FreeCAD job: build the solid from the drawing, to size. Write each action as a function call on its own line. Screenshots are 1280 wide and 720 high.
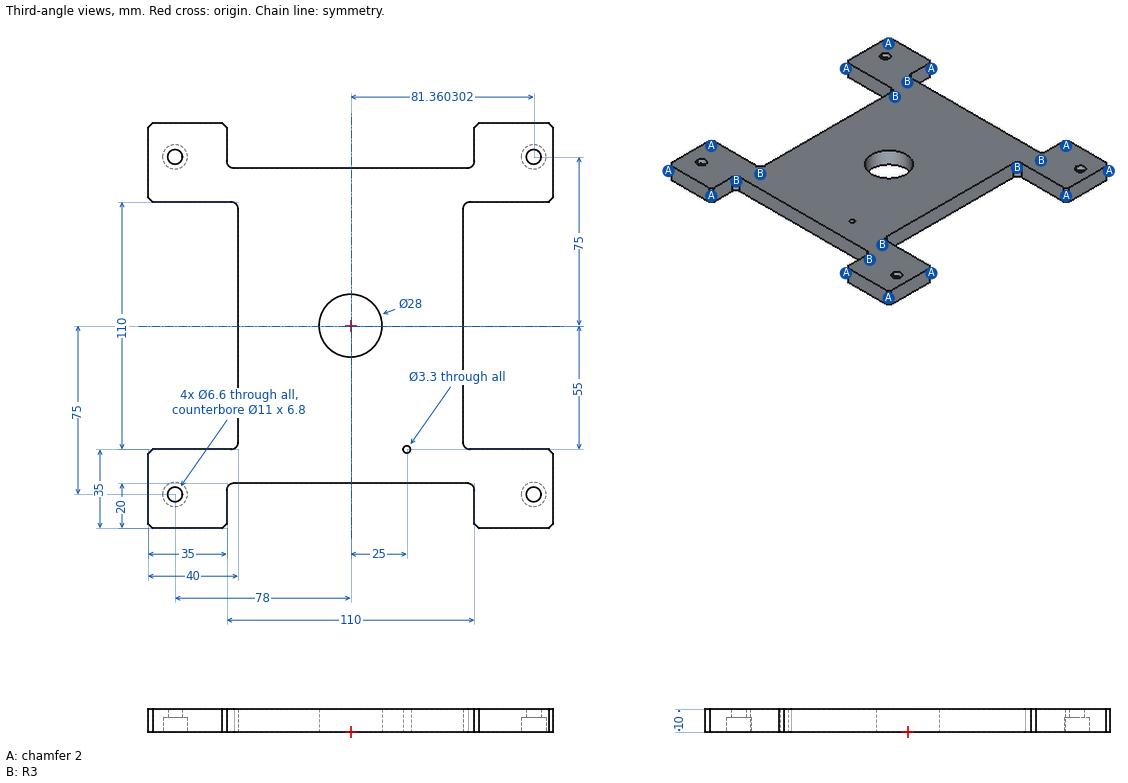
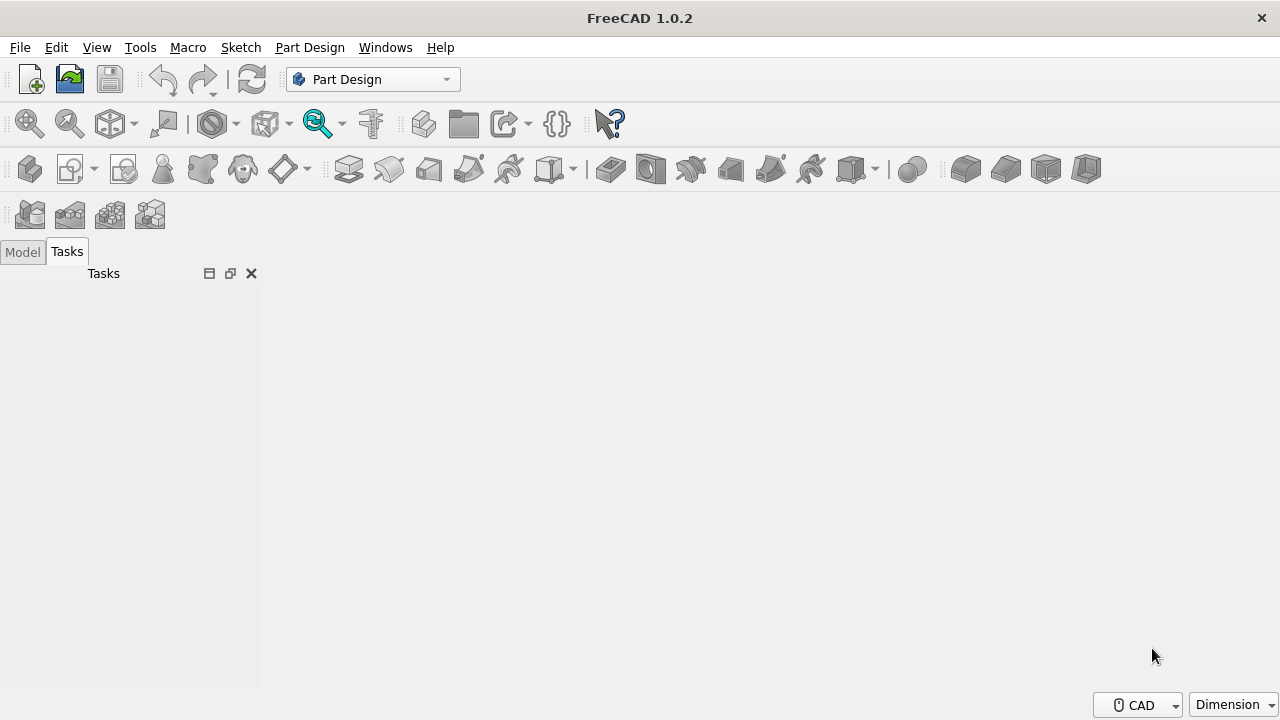
key(ctrl+n)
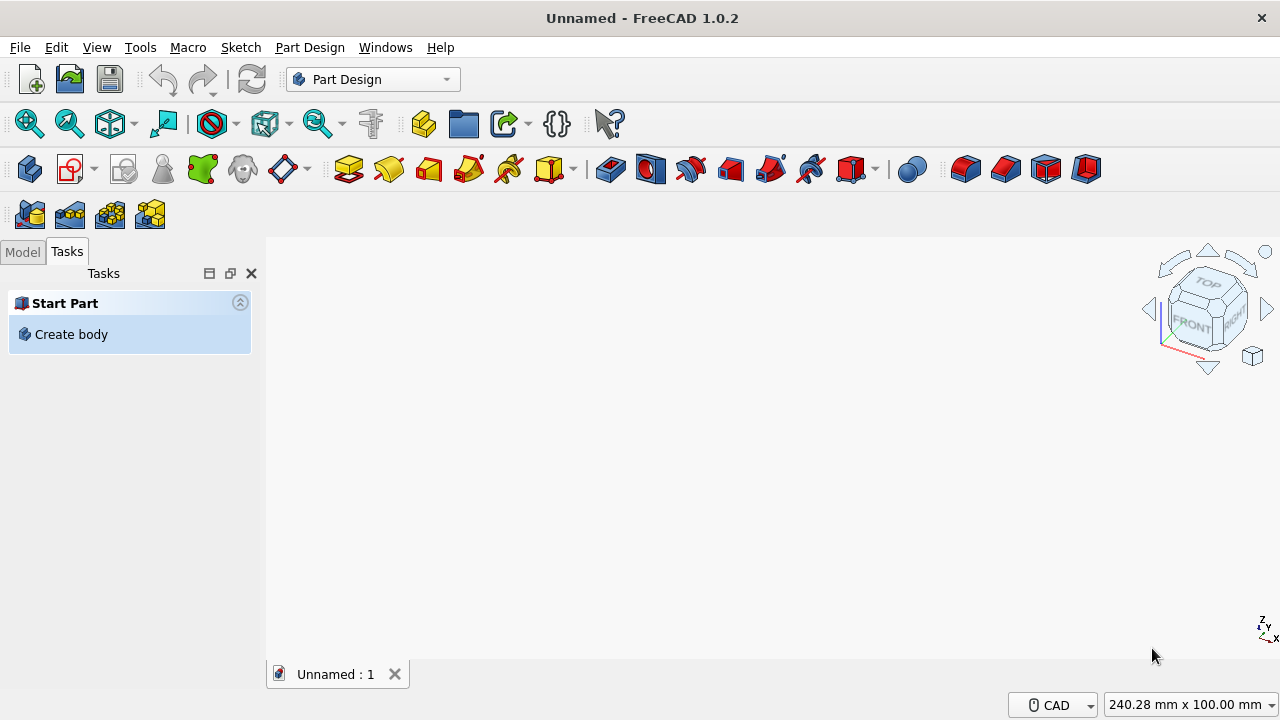
click(70, 170)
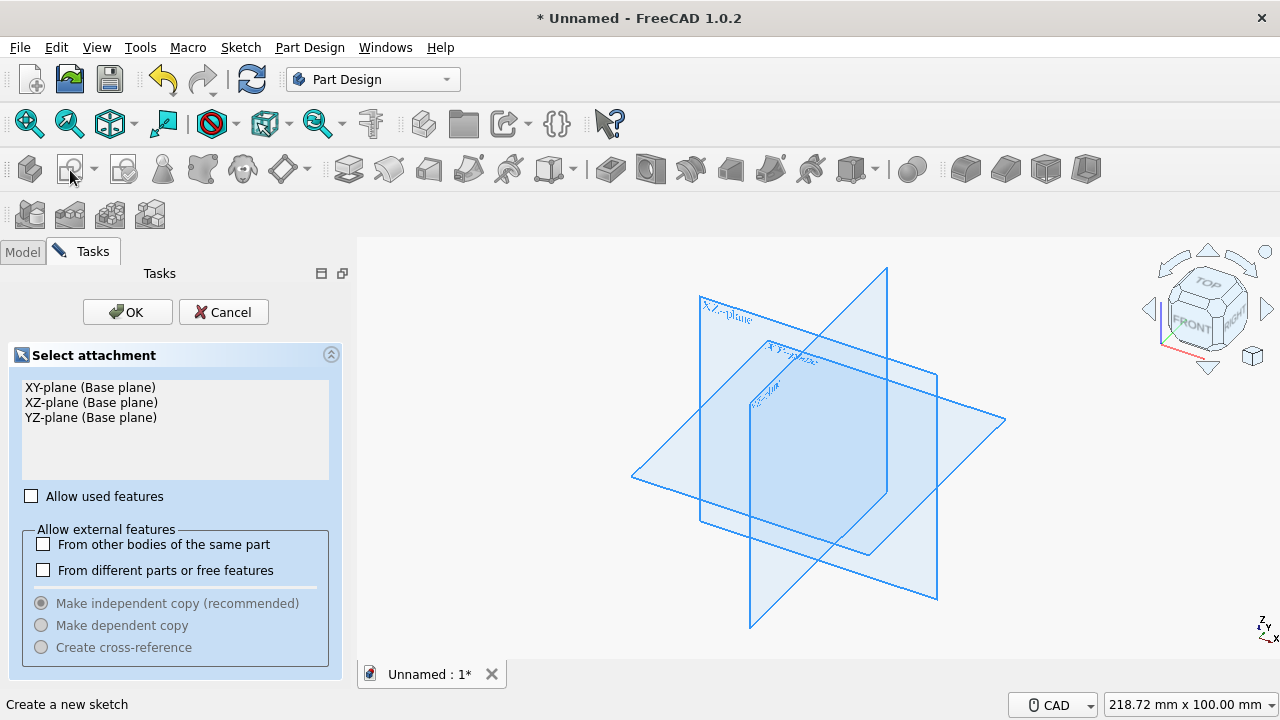
click(82, 388)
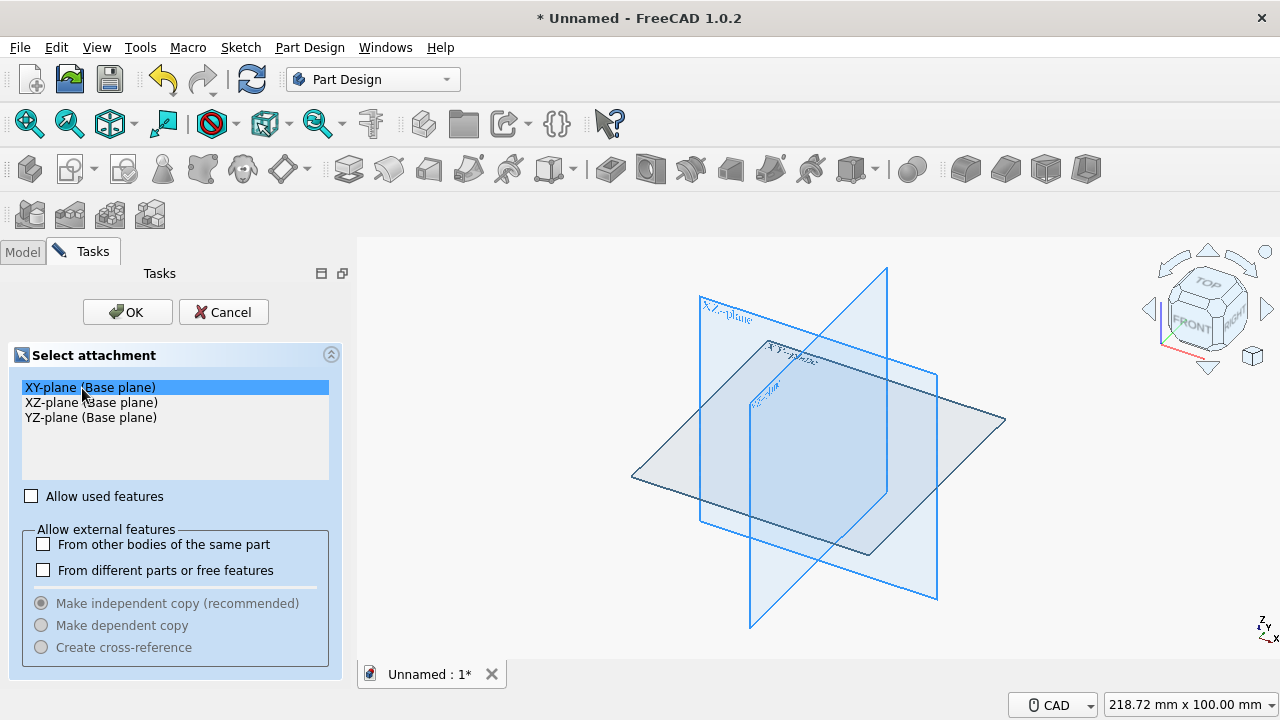
click(128, 312)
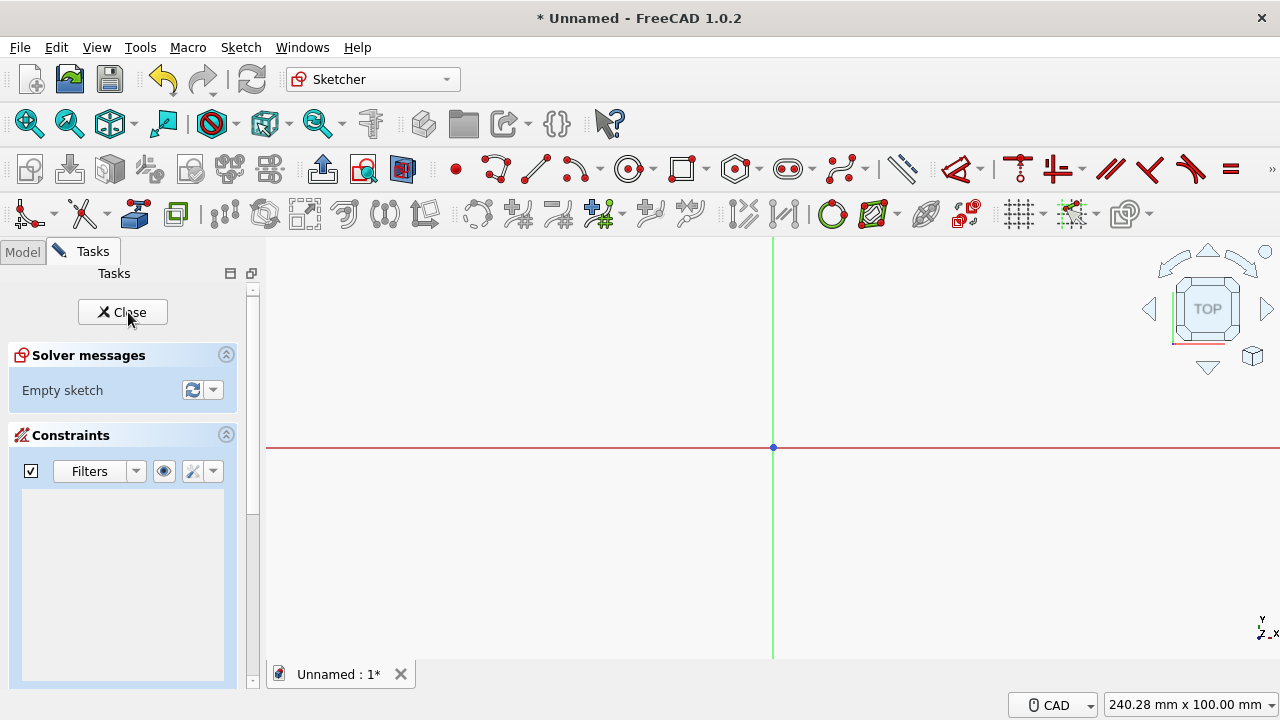
scroll(665, 448, down, 5)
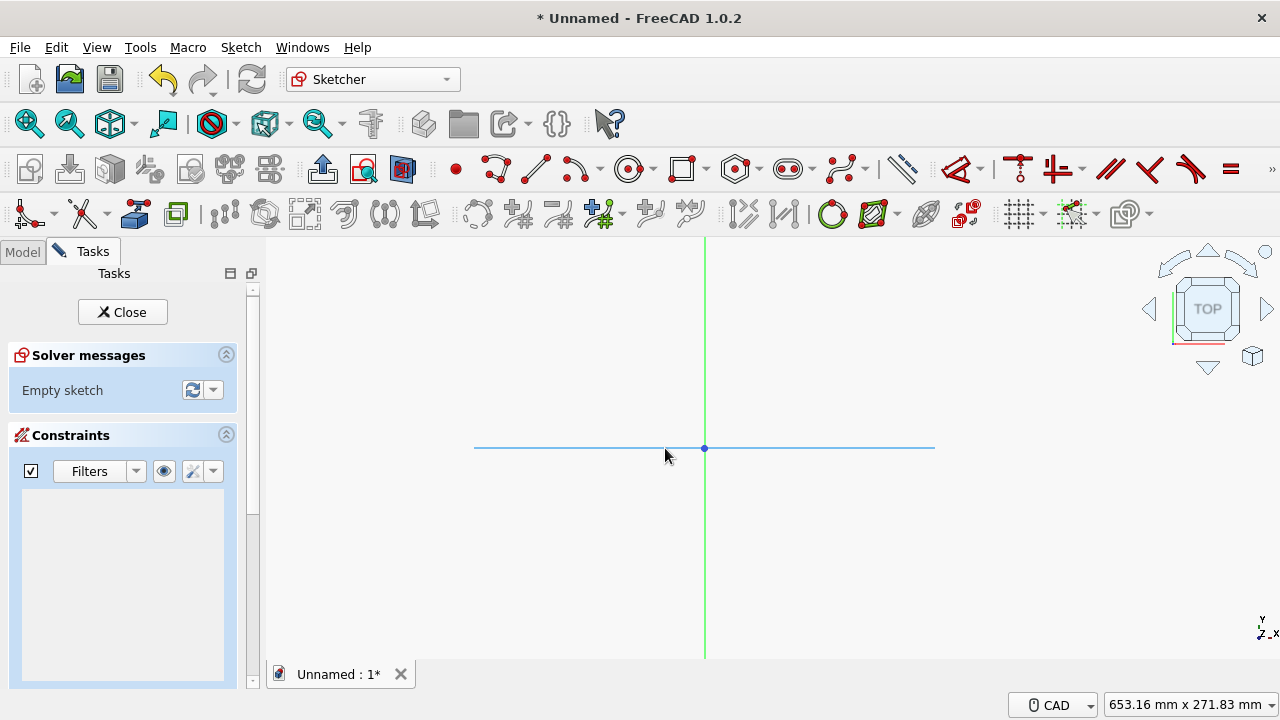
click(496, 170)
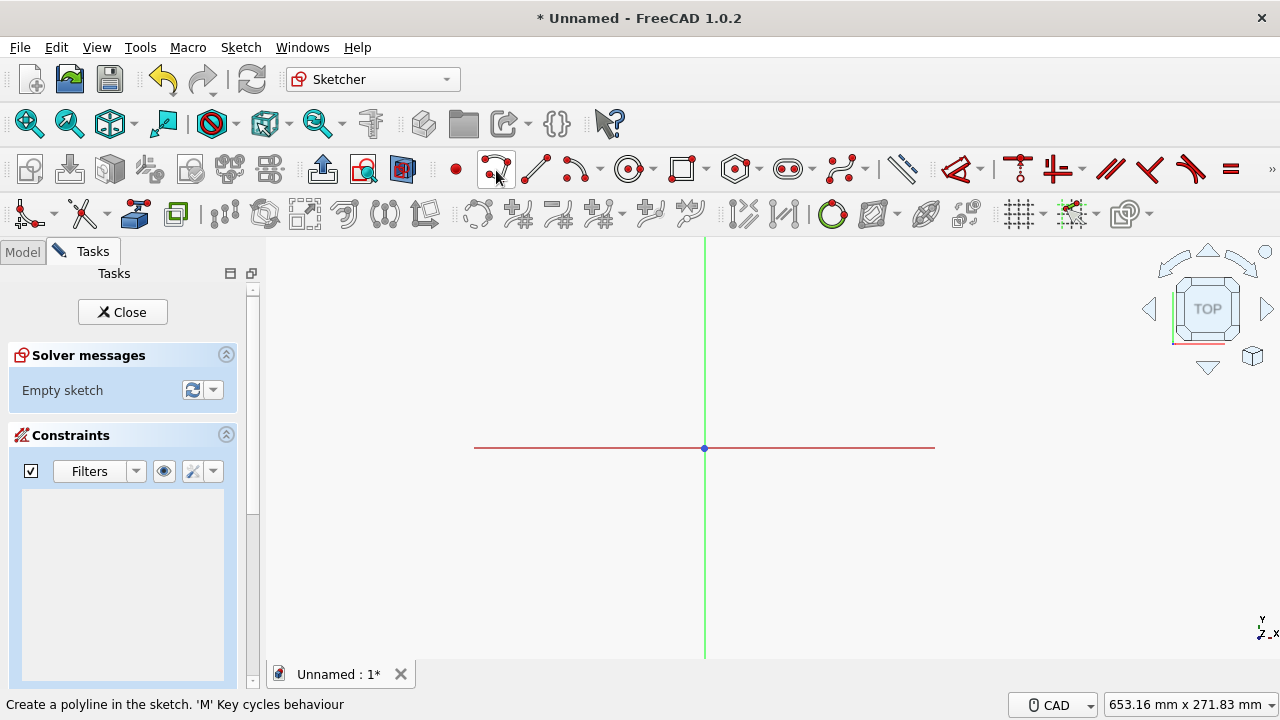
click(627, 363)
click(627, 534)
click(565, 534)
click(565, 588)
click(620, 588)
click(620, 557)
click(790, 557)
click(790, 588)
click(845, 588)
click(845, 534)
click(783, 534)
click(783, 363)
click(845, 363)
click(845, 309)
click(790, 309)
click(790, 340)
click(620, 340)
click(620, 309)
click(565, 309)
click(565, 363)
click(627, 364)
key(Escape)
key(Escape)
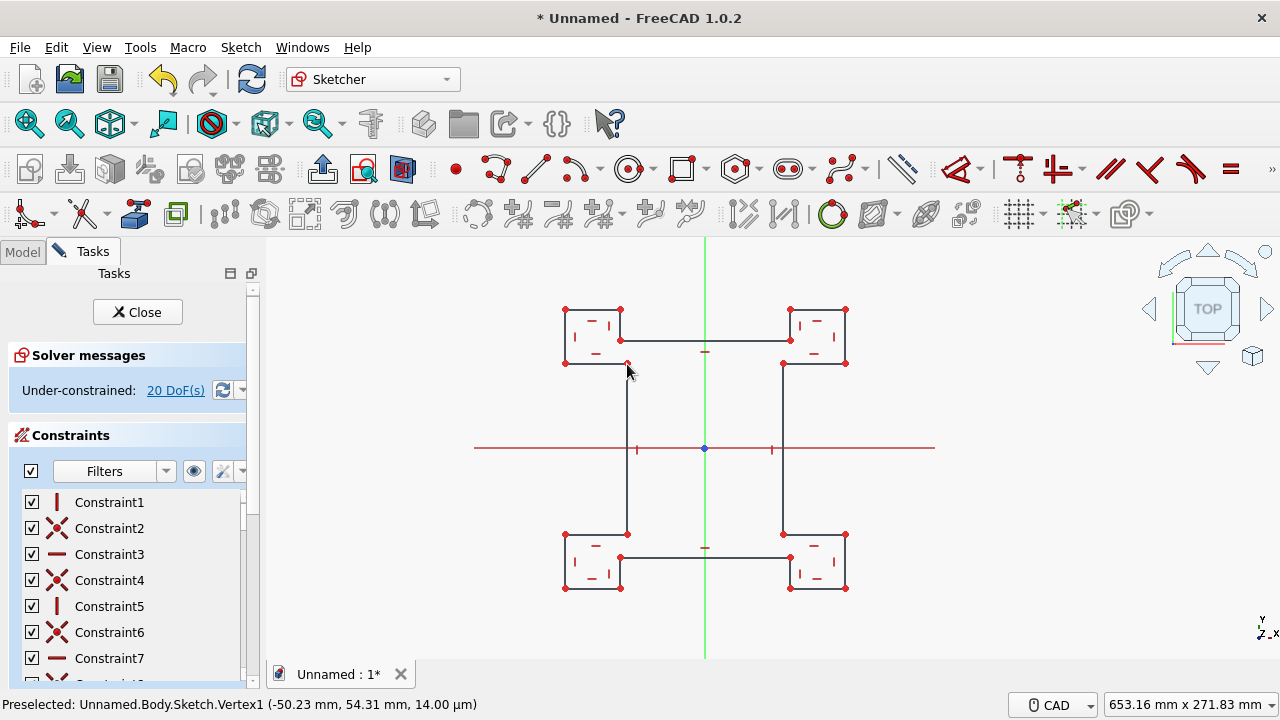
click(620, 589)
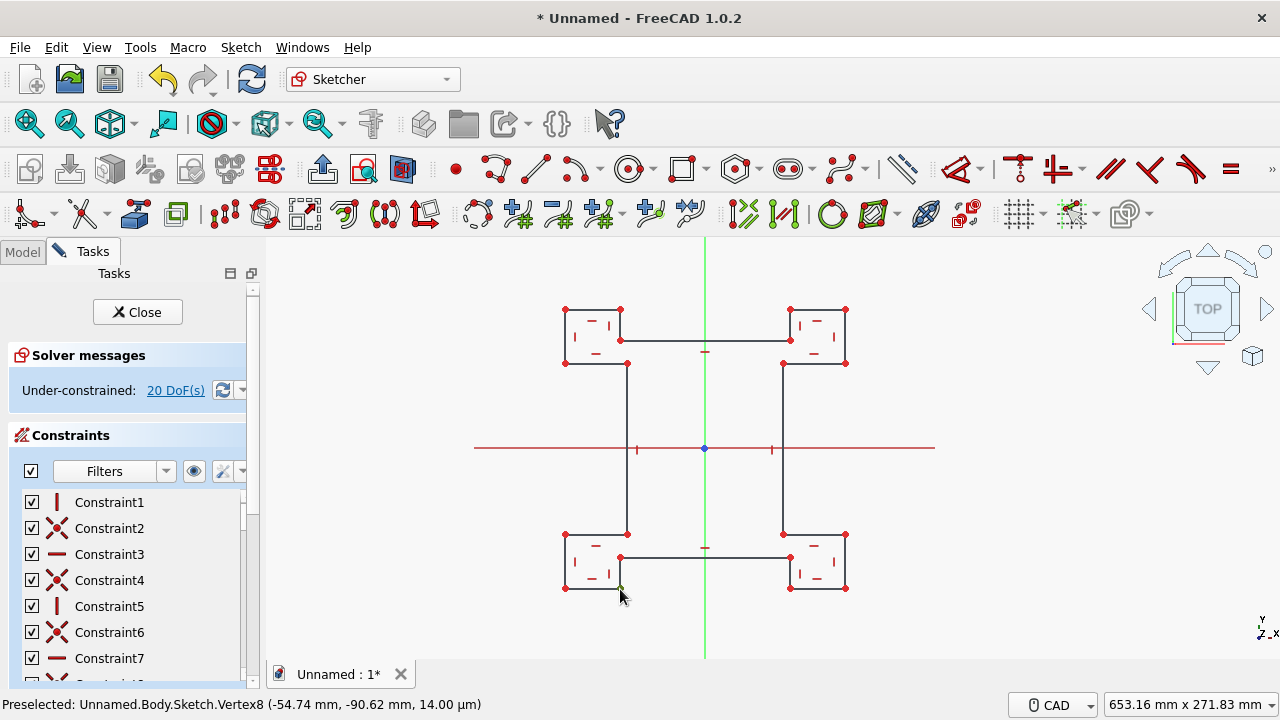
click(790, 589)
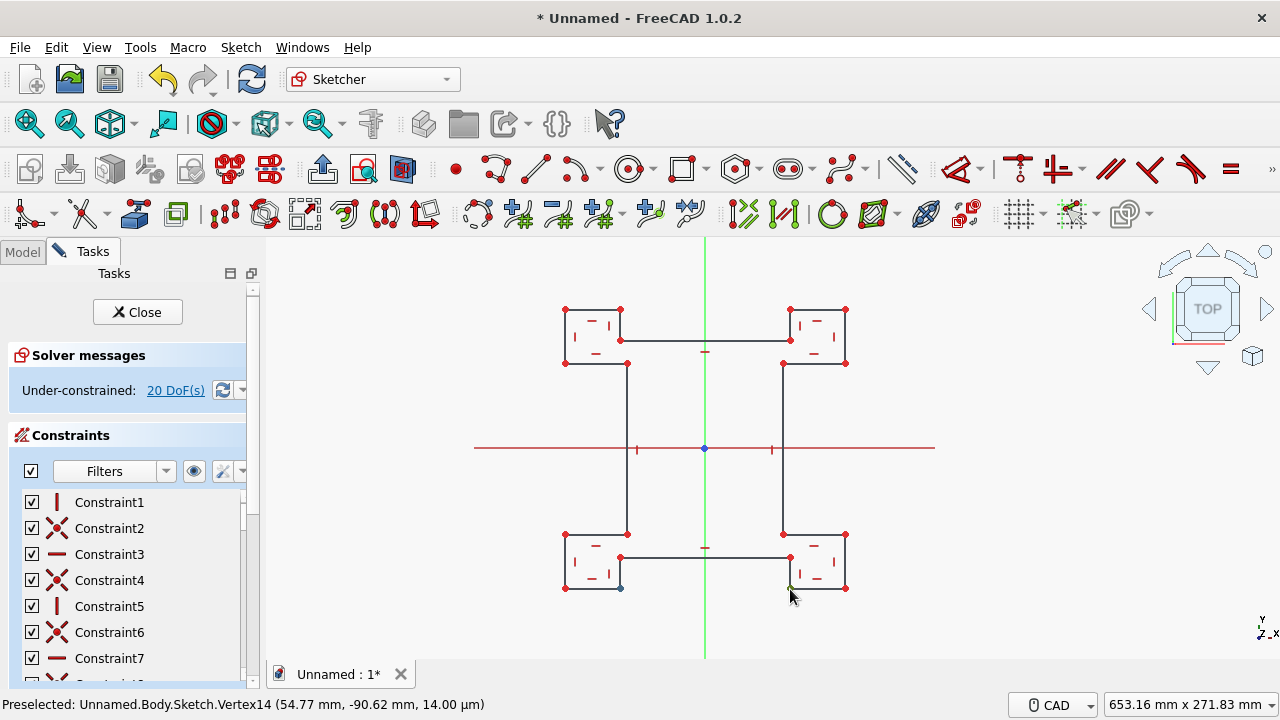
click(705, 605)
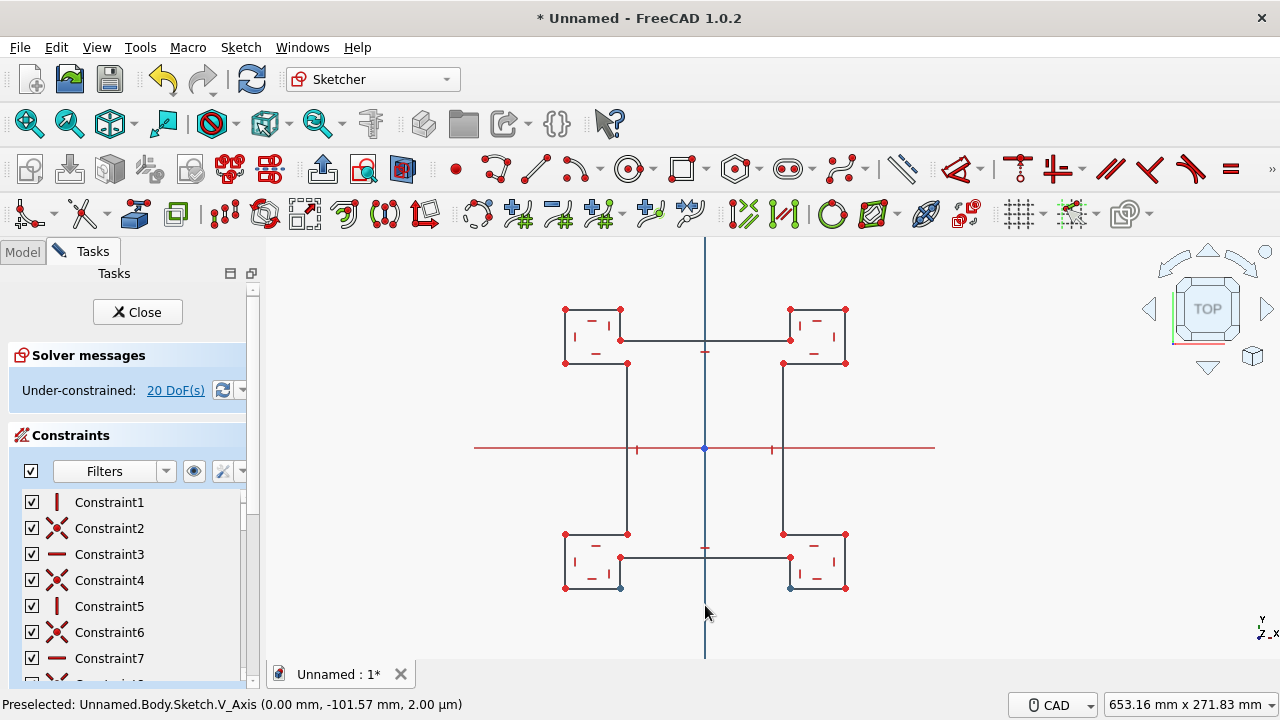
key(s)